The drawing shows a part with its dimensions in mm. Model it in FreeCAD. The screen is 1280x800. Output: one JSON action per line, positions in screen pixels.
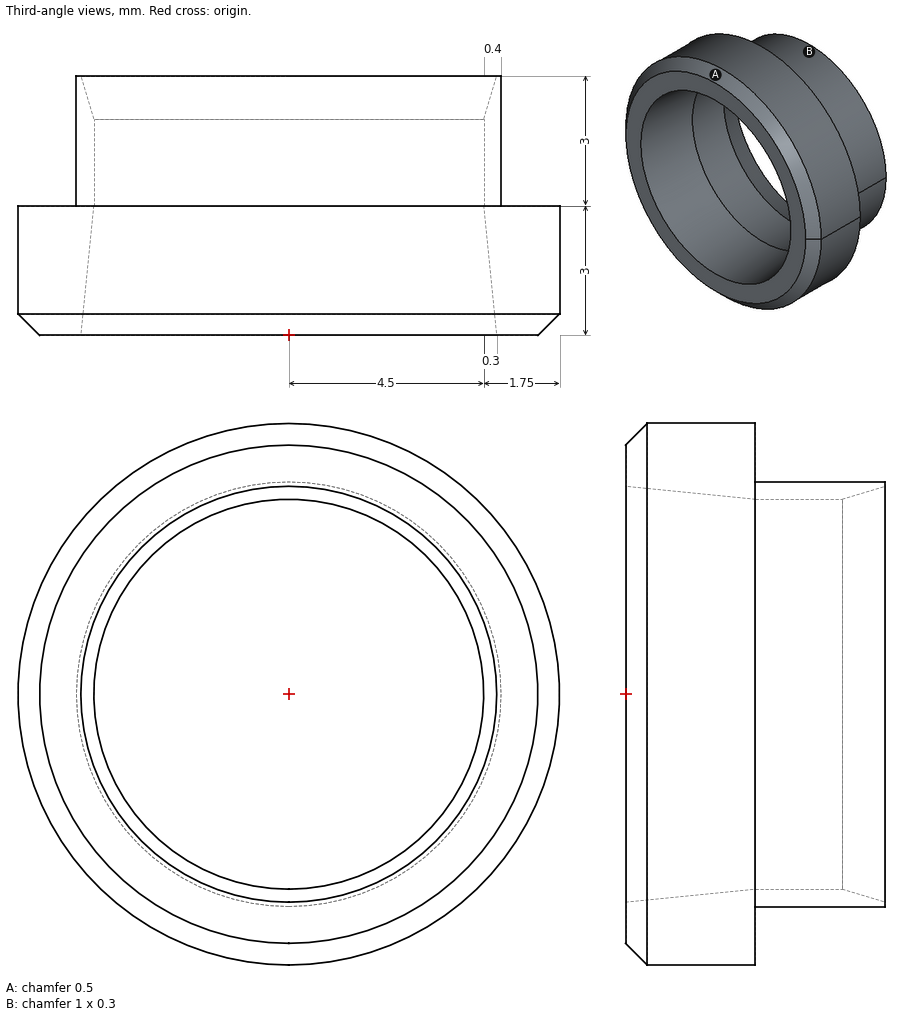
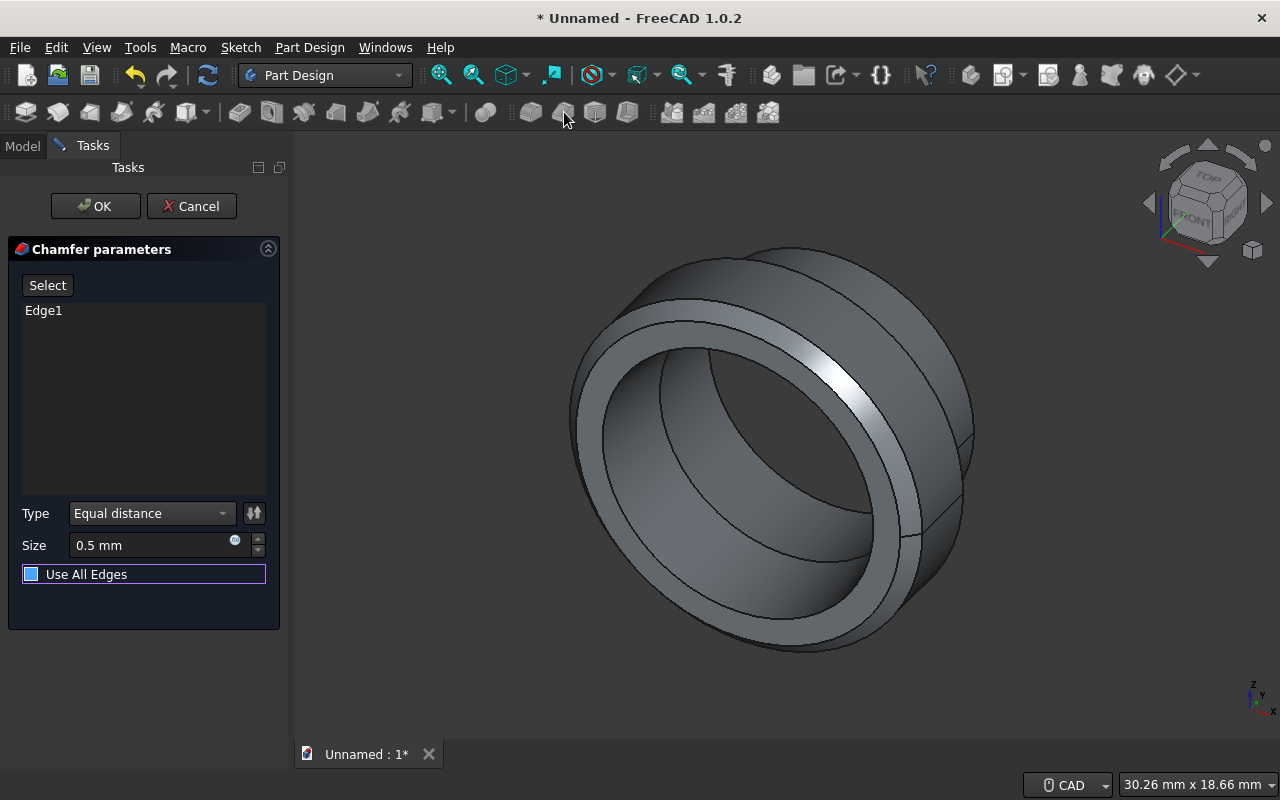
{"action": "left_click", "coordinate": [96, 206]}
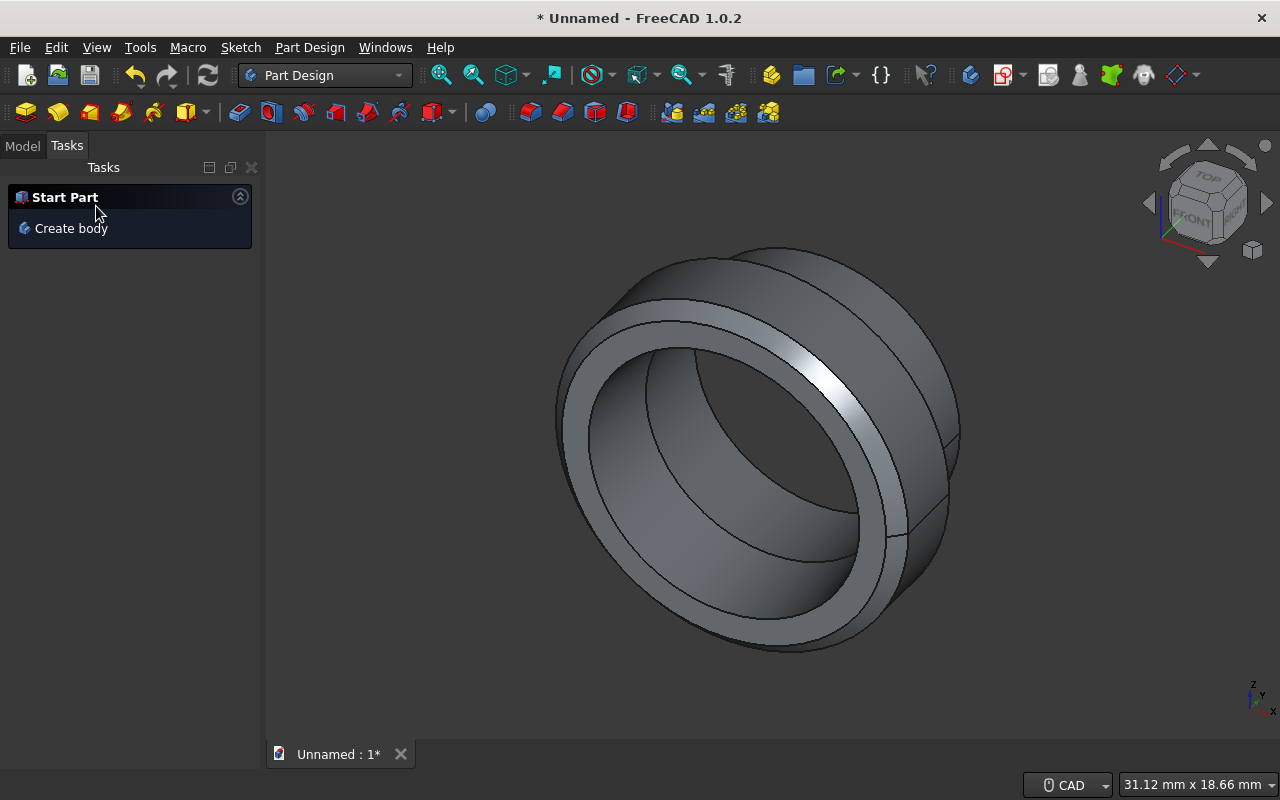
{"action": "key", "text": "0"}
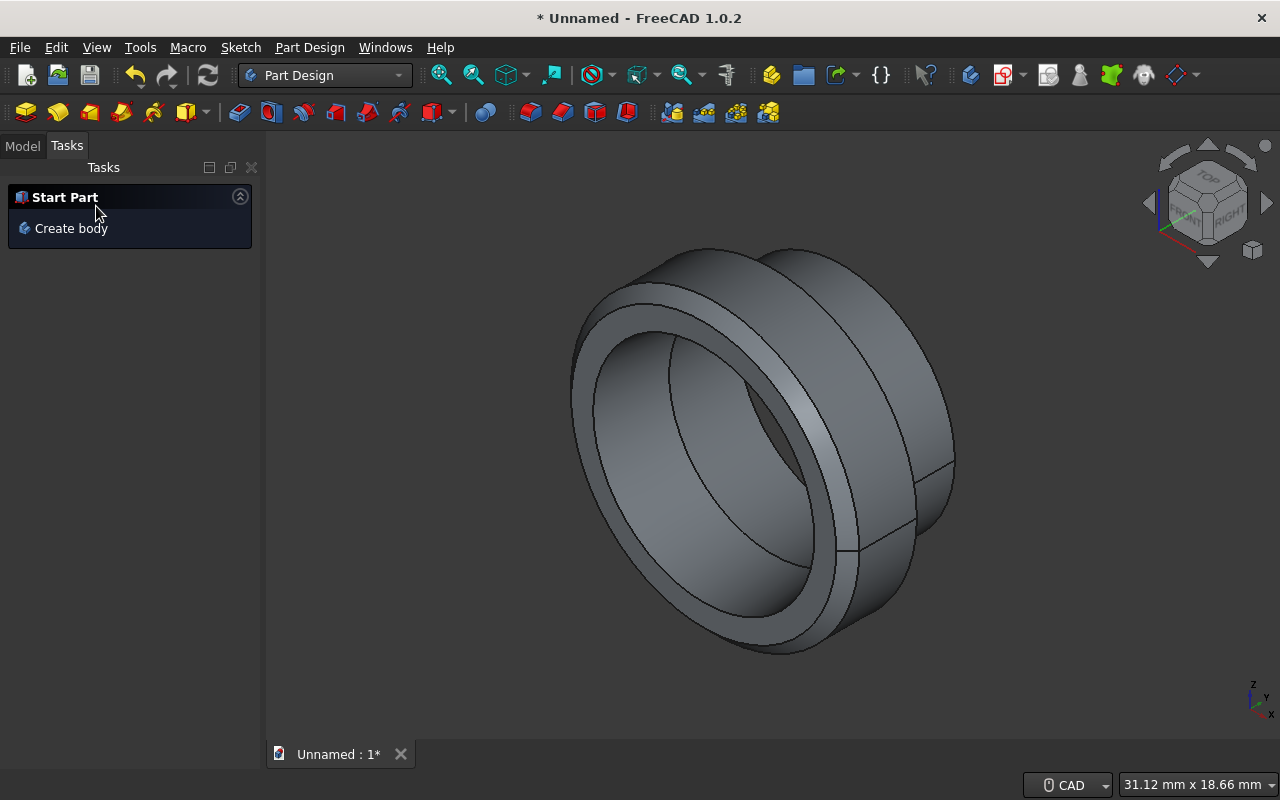
{"action": "key", "text": "2"}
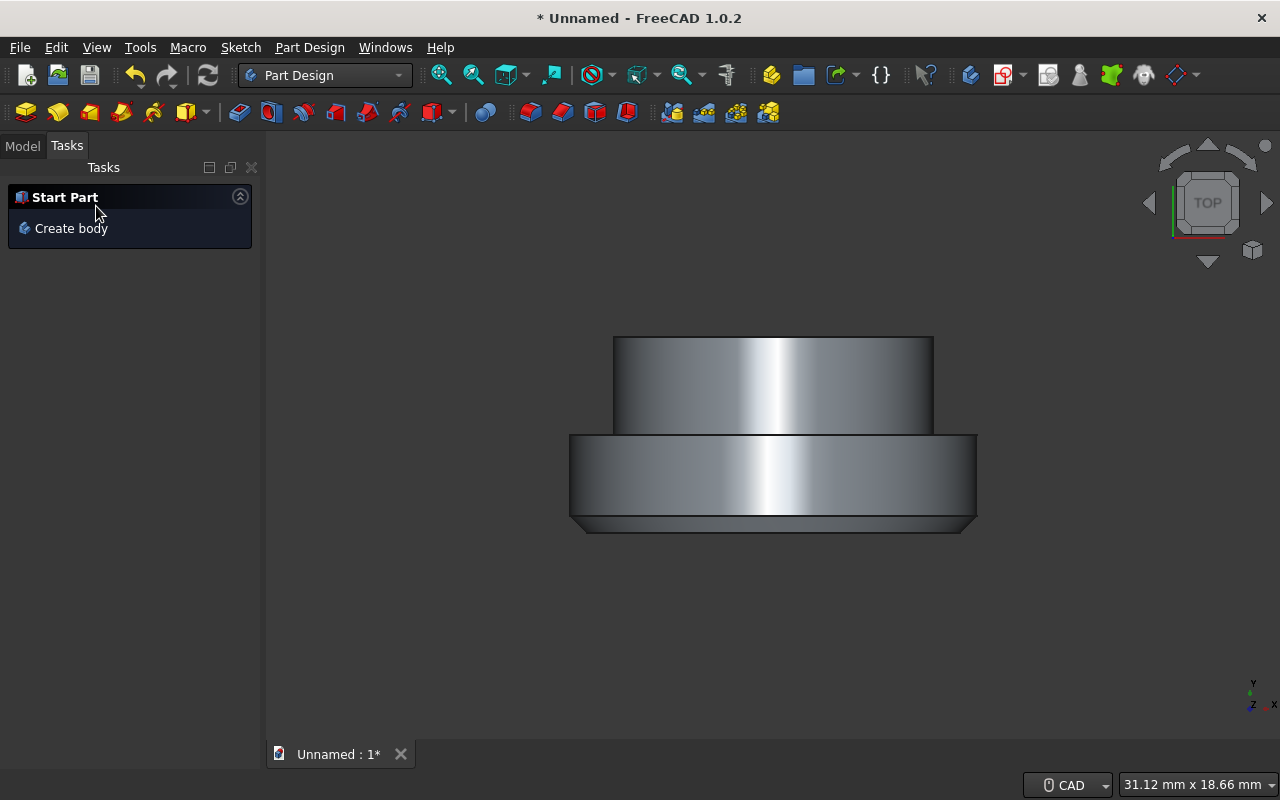
{"action": "left_click", "coordinate": [442, 76]}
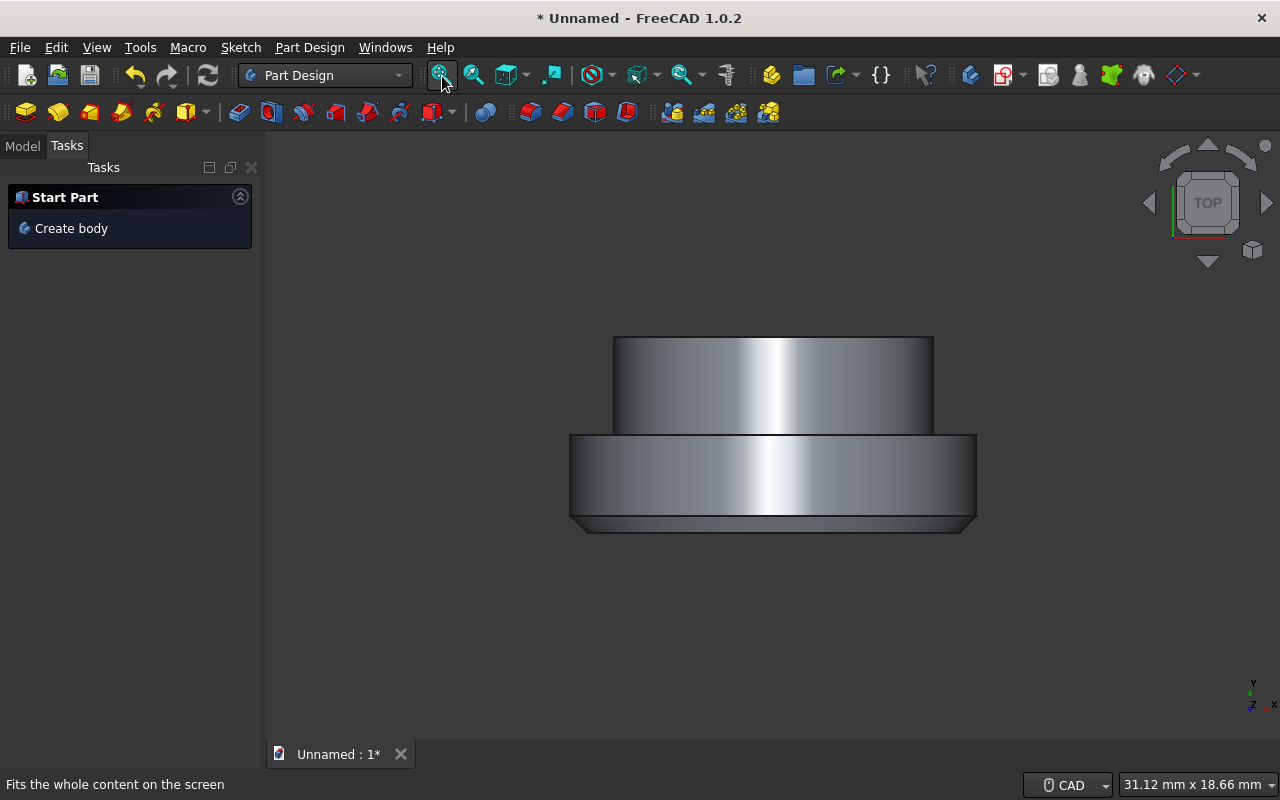
{"action": "key", "text": "1"}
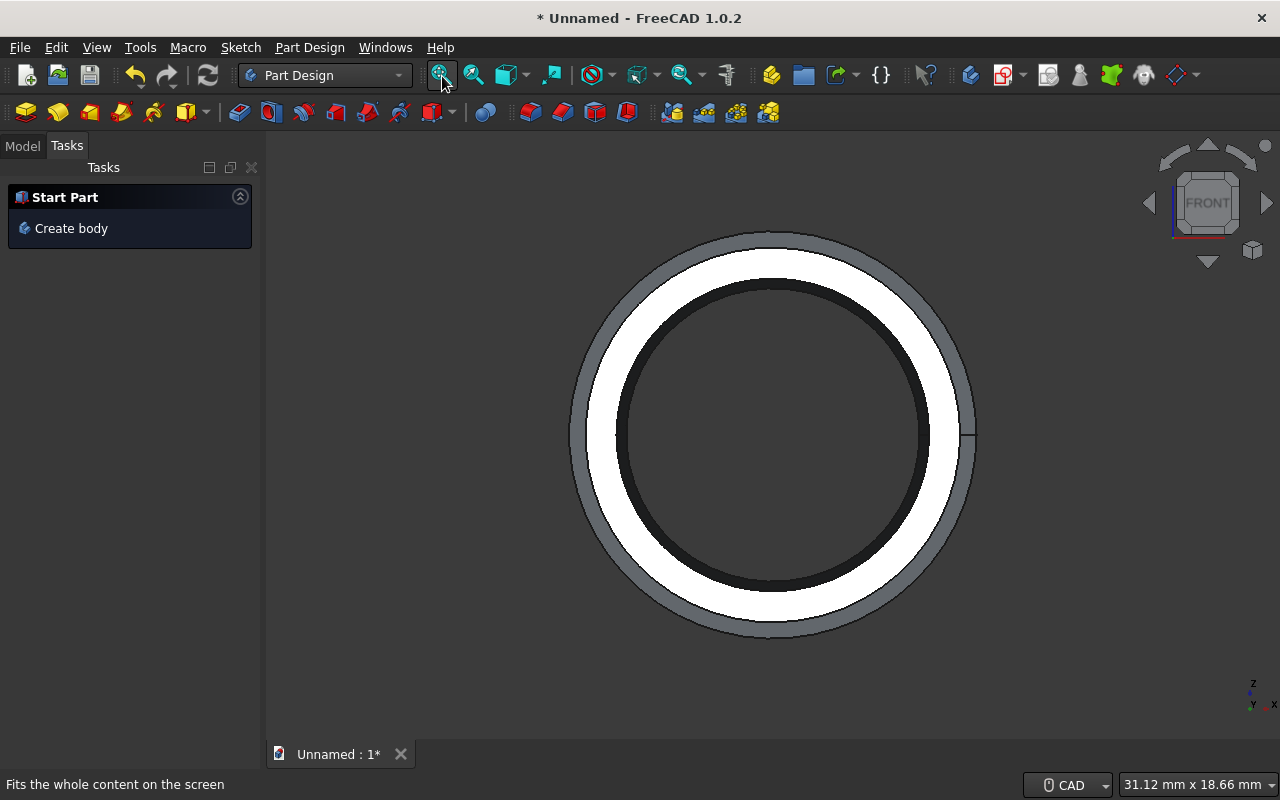
{"action": "key", "text": "3"}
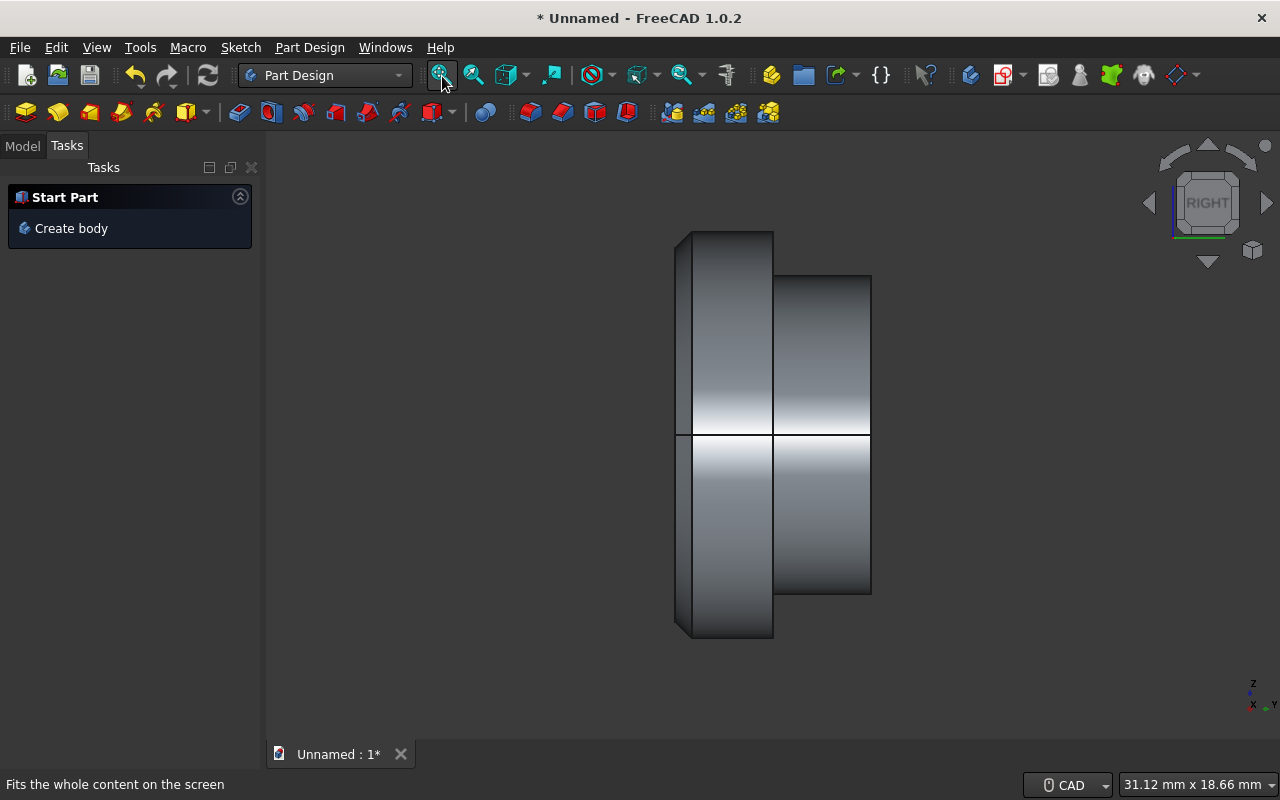
{"action": "key", "text": "5"}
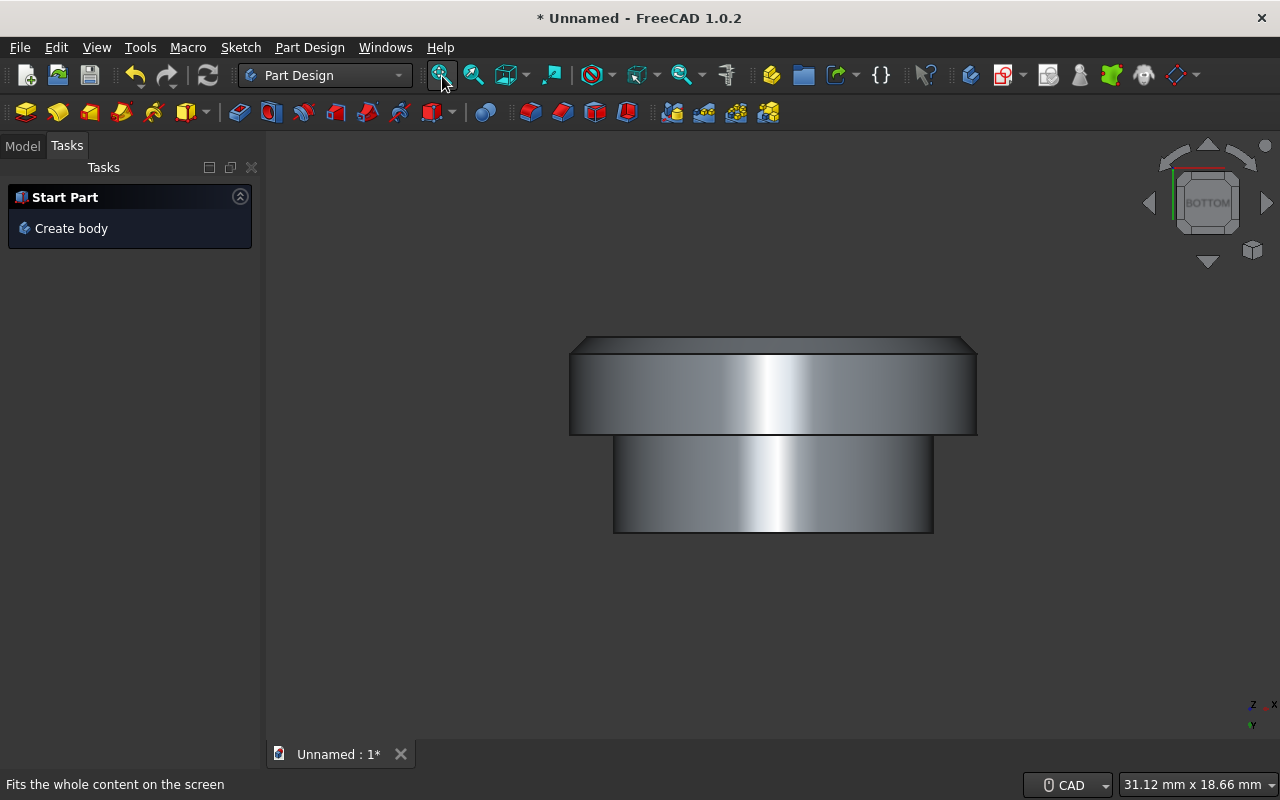
{"action": "left_click", "coordinate": [442, 76]}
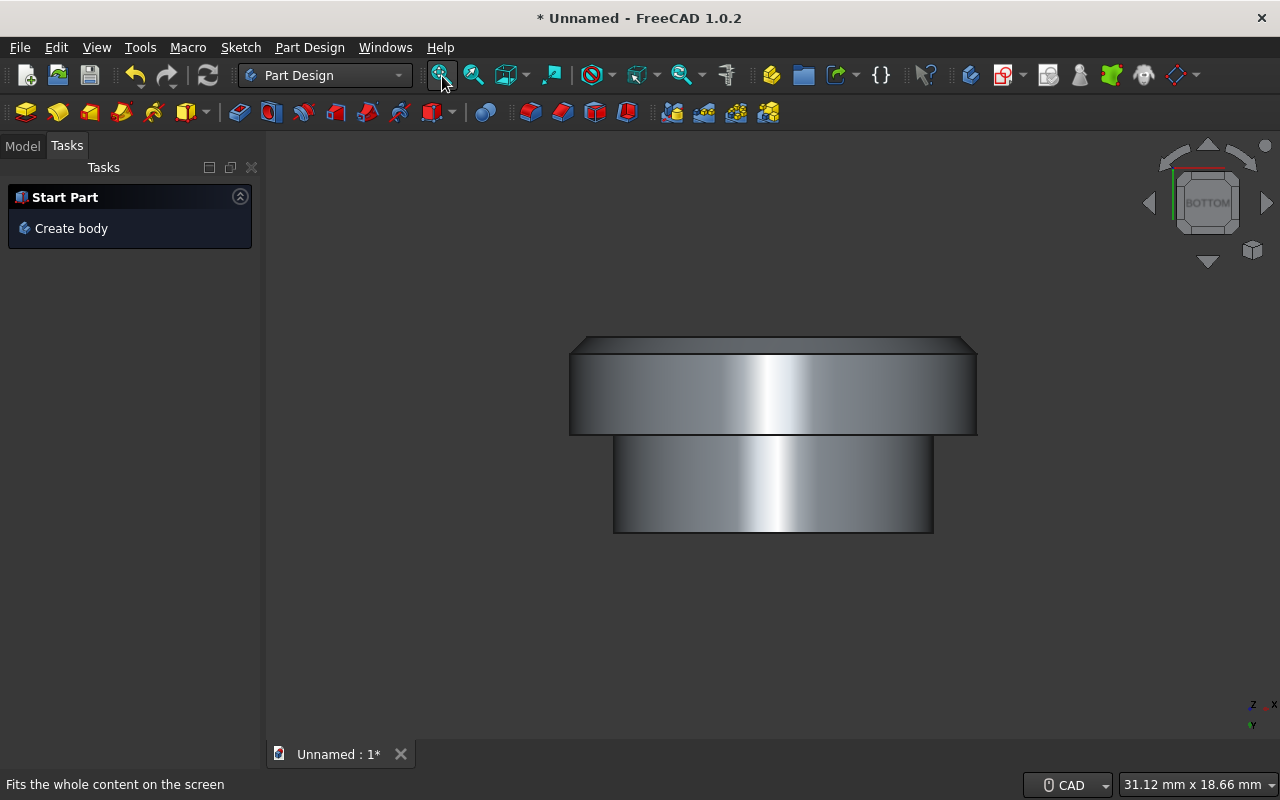
{"action": "key", "text": "4"}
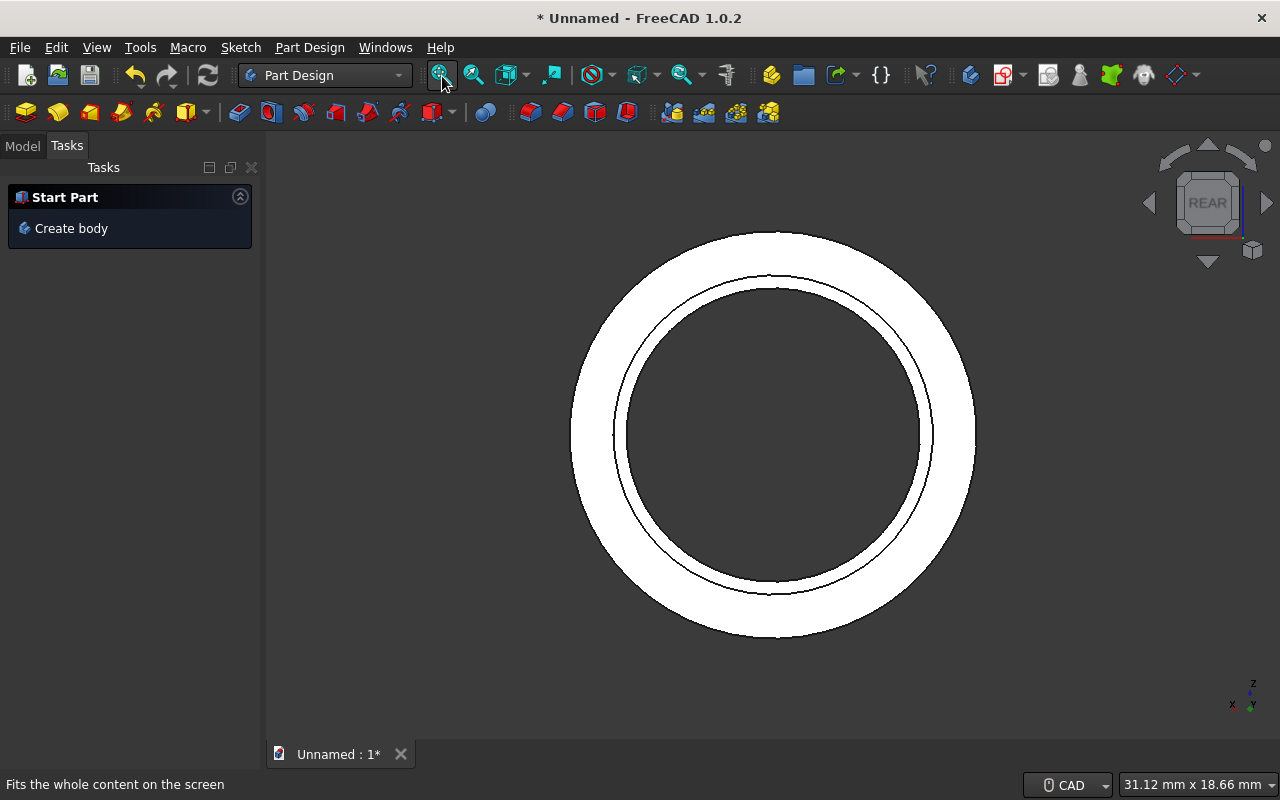
{"action": "left_click", "coordinate": [920, 434]}